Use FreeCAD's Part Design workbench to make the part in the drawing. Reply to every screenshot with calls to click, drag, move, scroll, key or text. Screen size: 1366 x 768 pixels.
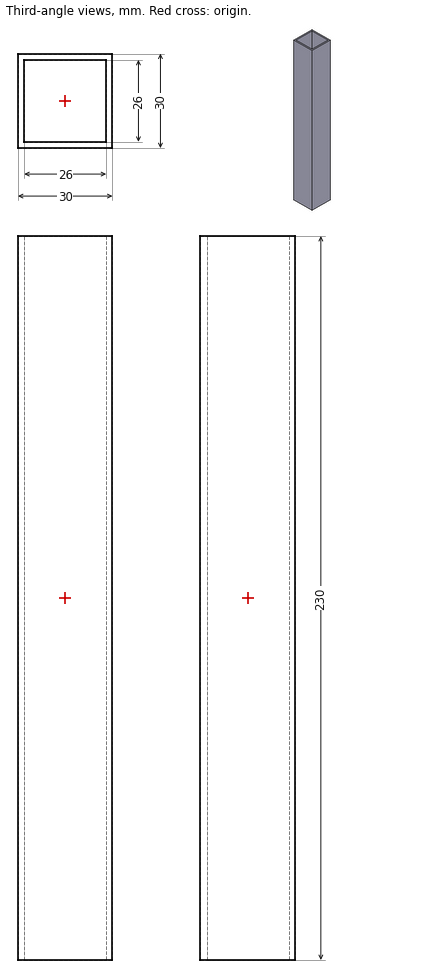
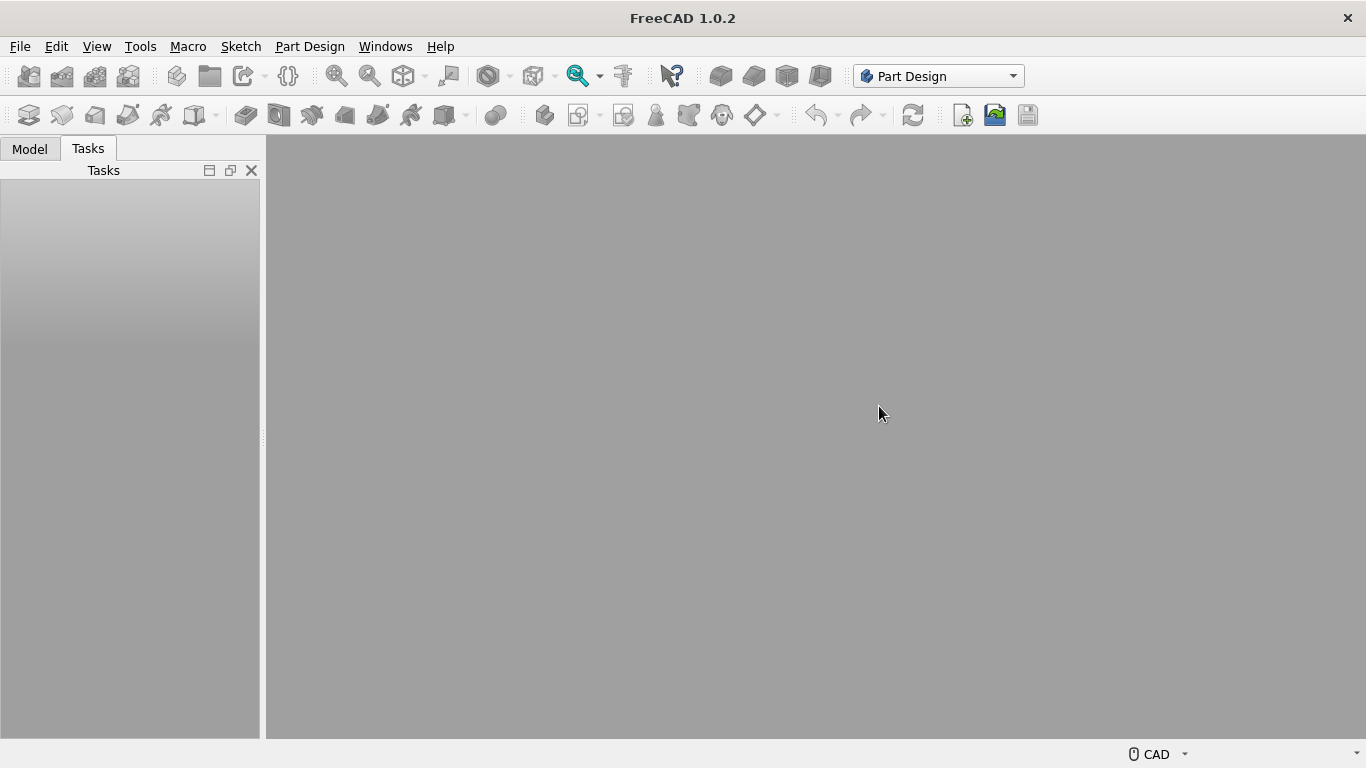
key(ctrl+n)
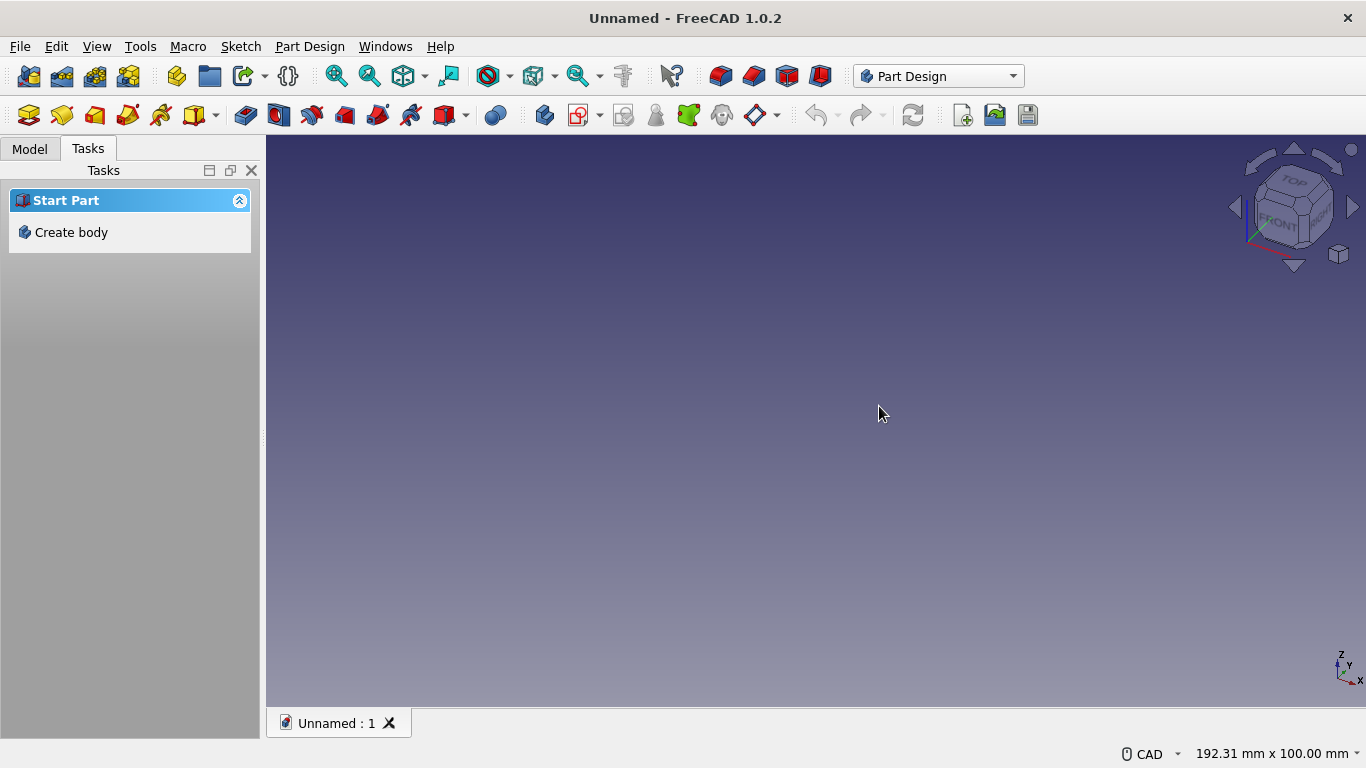
click(578, 116)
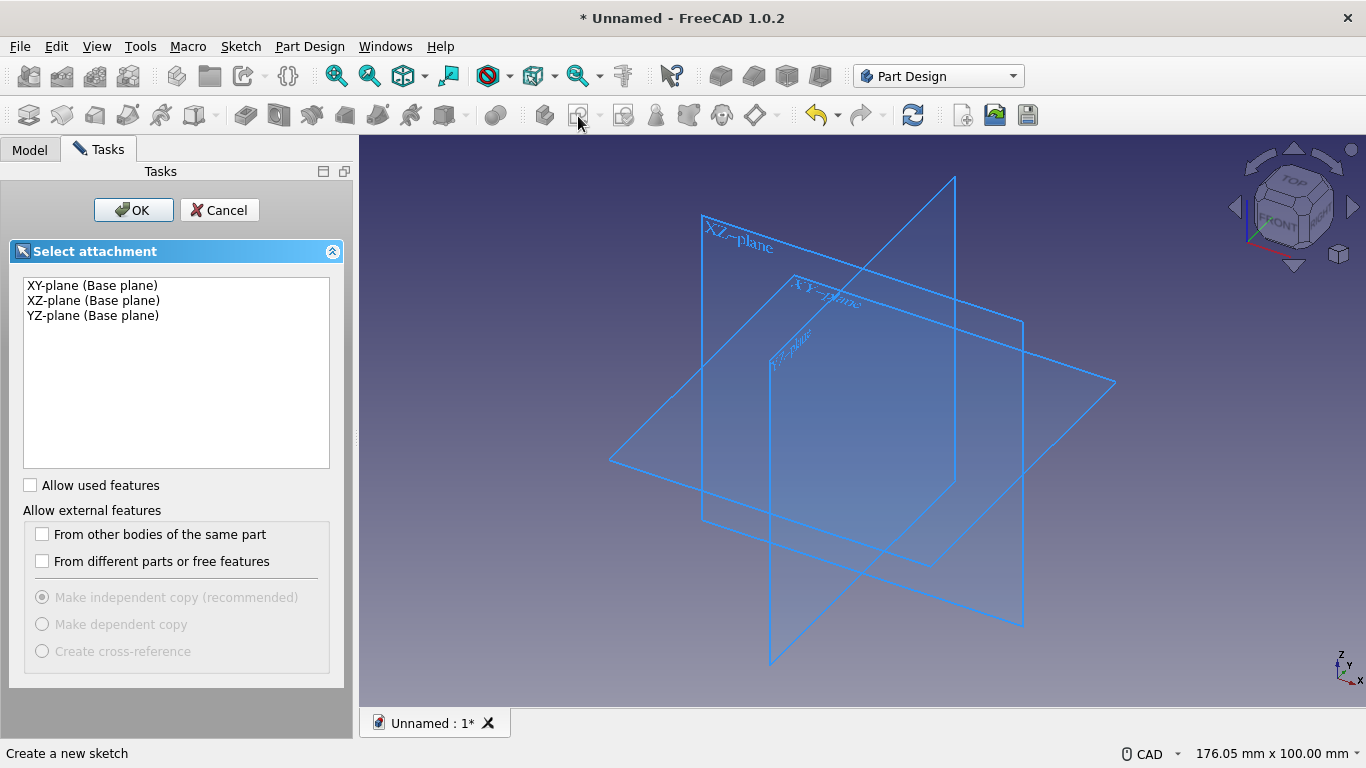
click(84, 286)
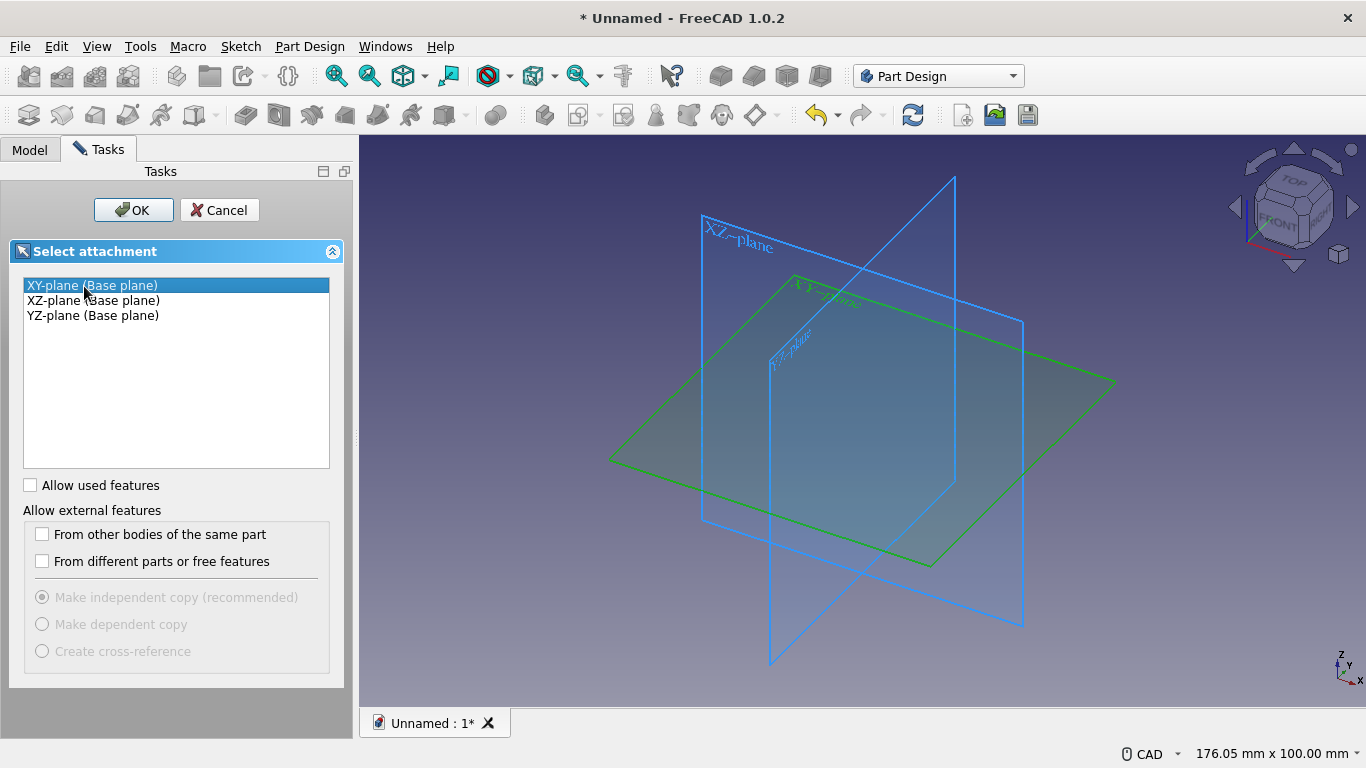
click(134, 210)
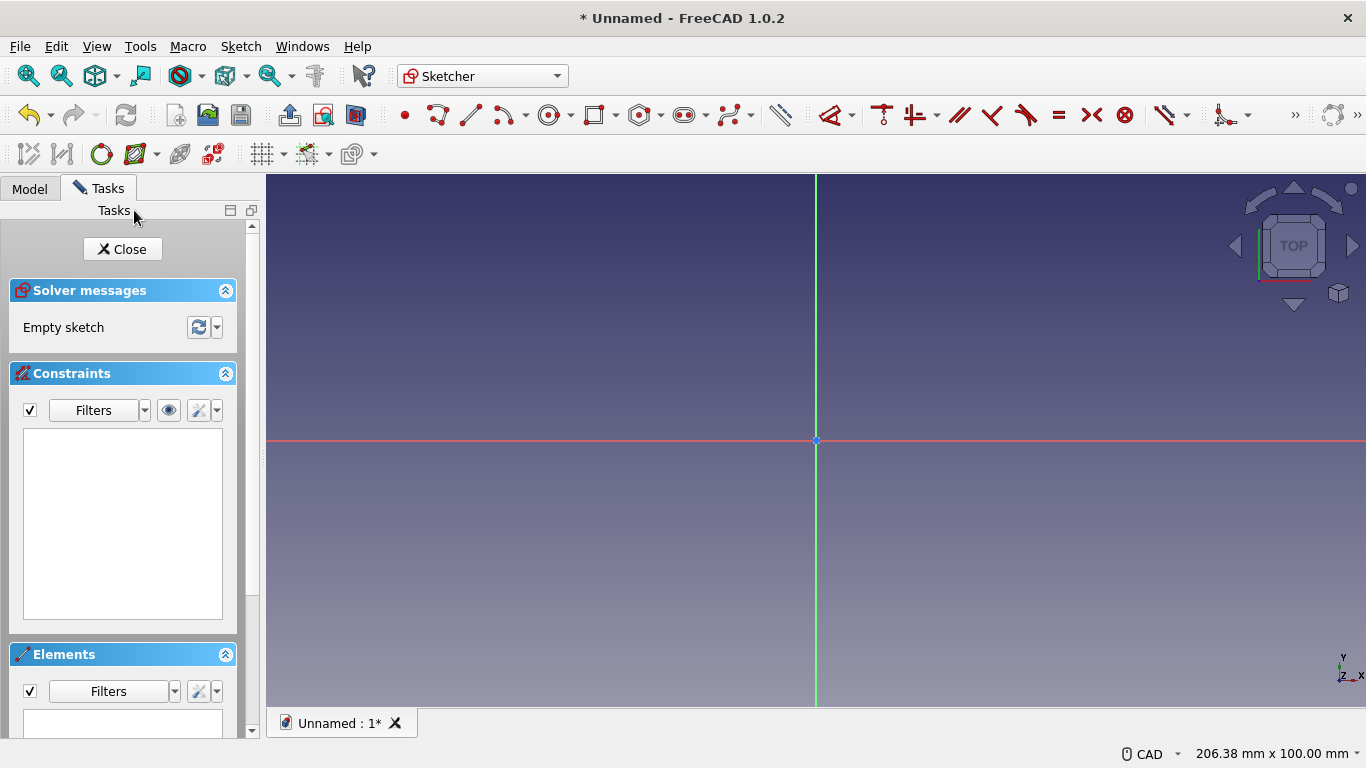
scroll(872, 440, up, 4)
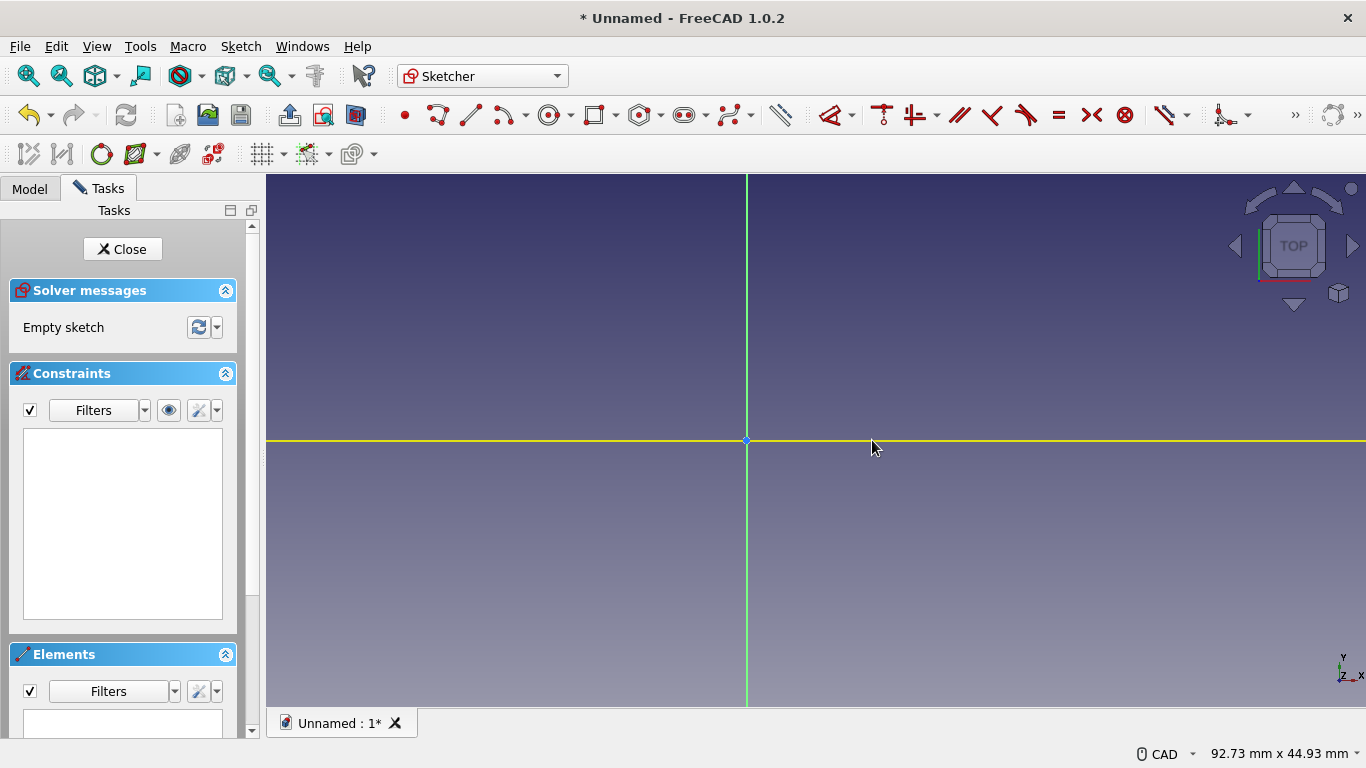
key(g)
key(v)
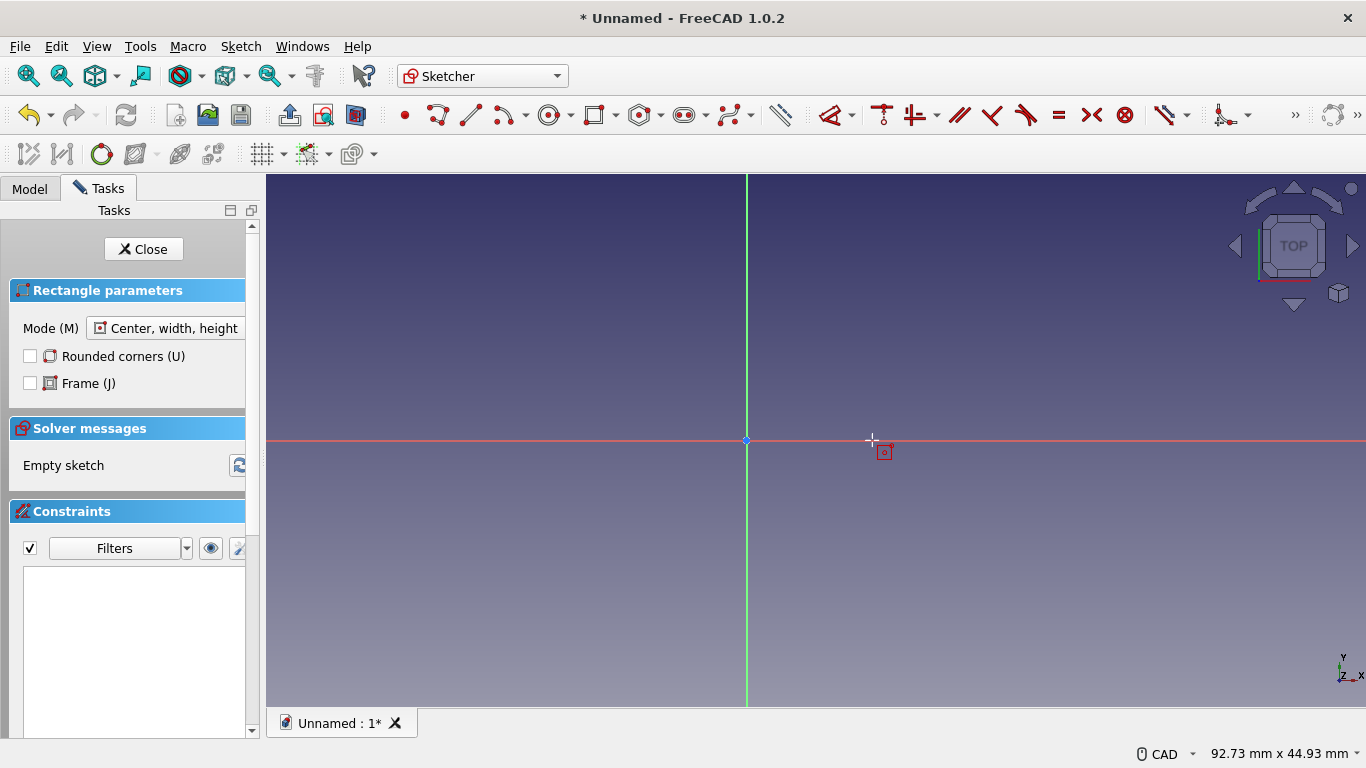
click(747, 440)
move(925, 263)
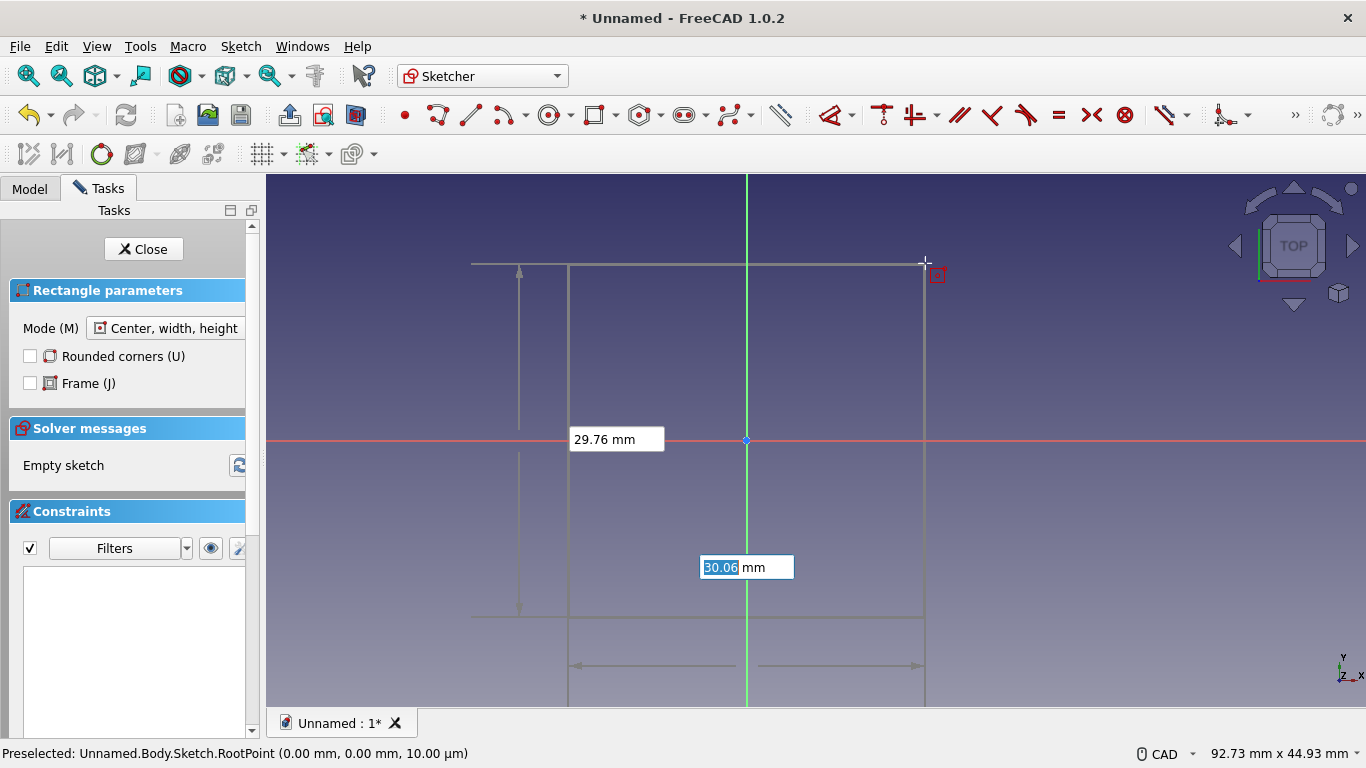
text(30)
key(Tab)
text(30)
key(Return)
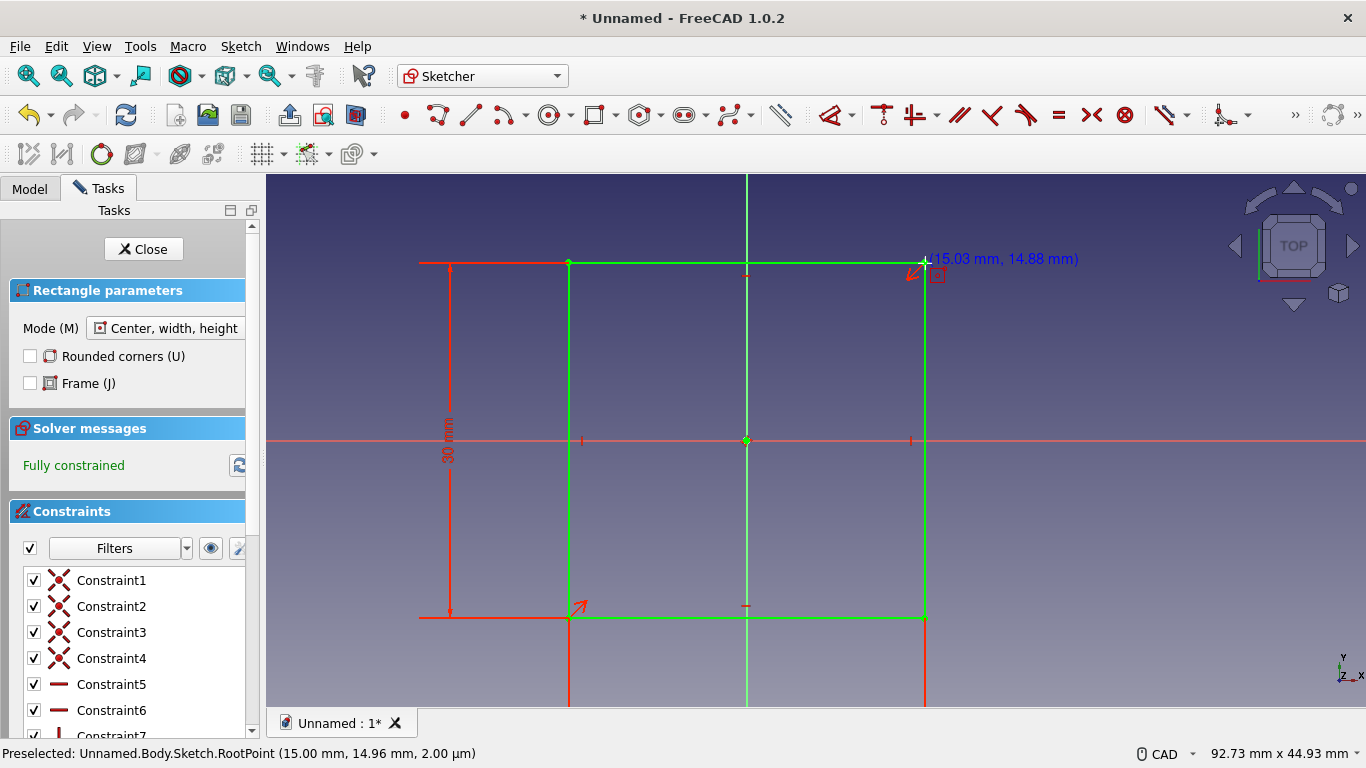
click(747, 440)
move(901, 286)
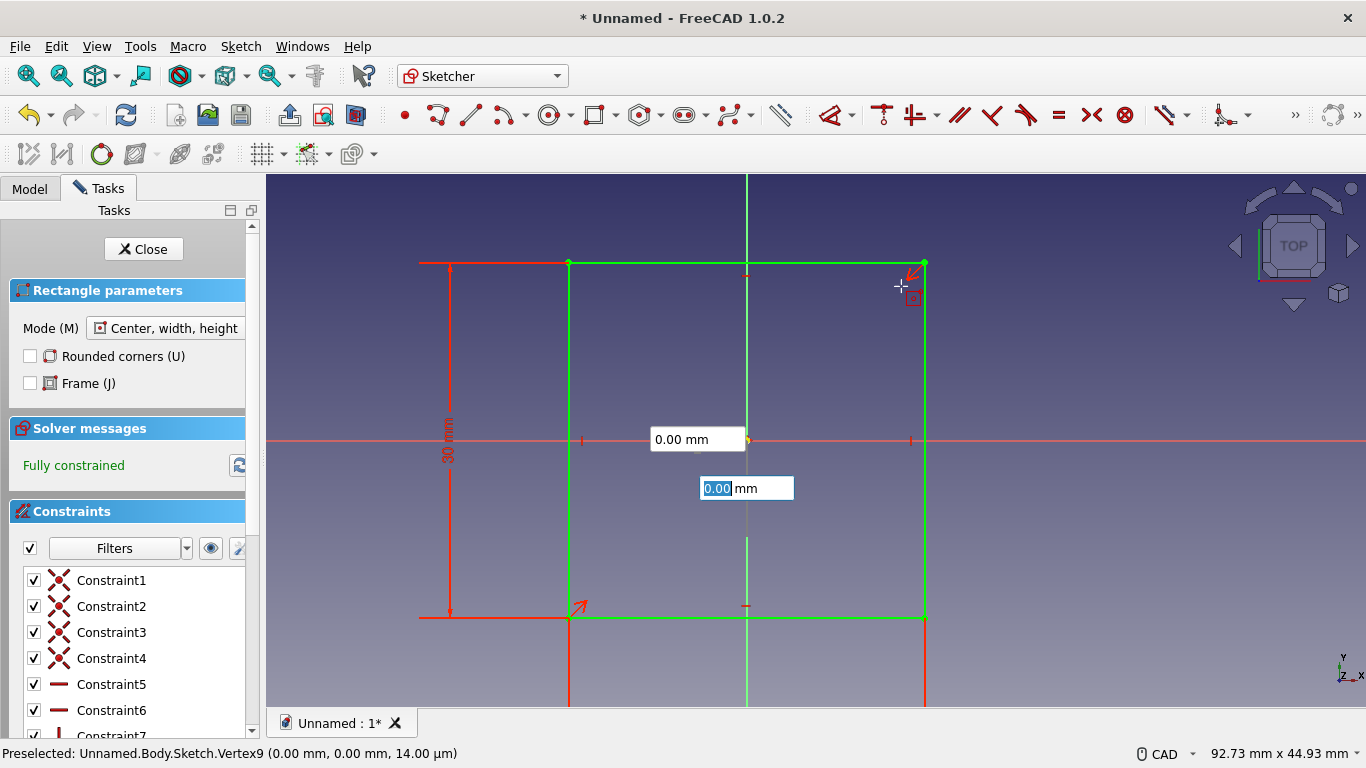
text(26)
key(Tab)
text(26)
key(Return)
key(Escape)